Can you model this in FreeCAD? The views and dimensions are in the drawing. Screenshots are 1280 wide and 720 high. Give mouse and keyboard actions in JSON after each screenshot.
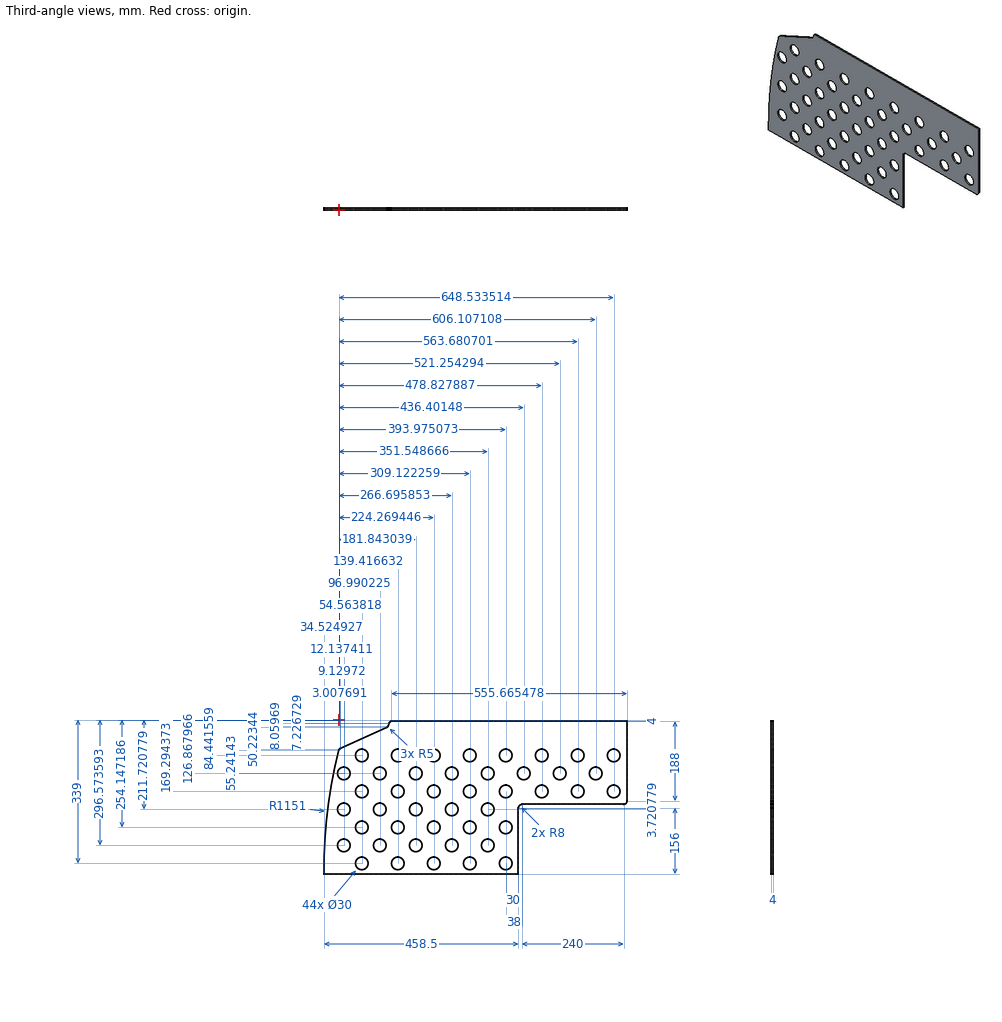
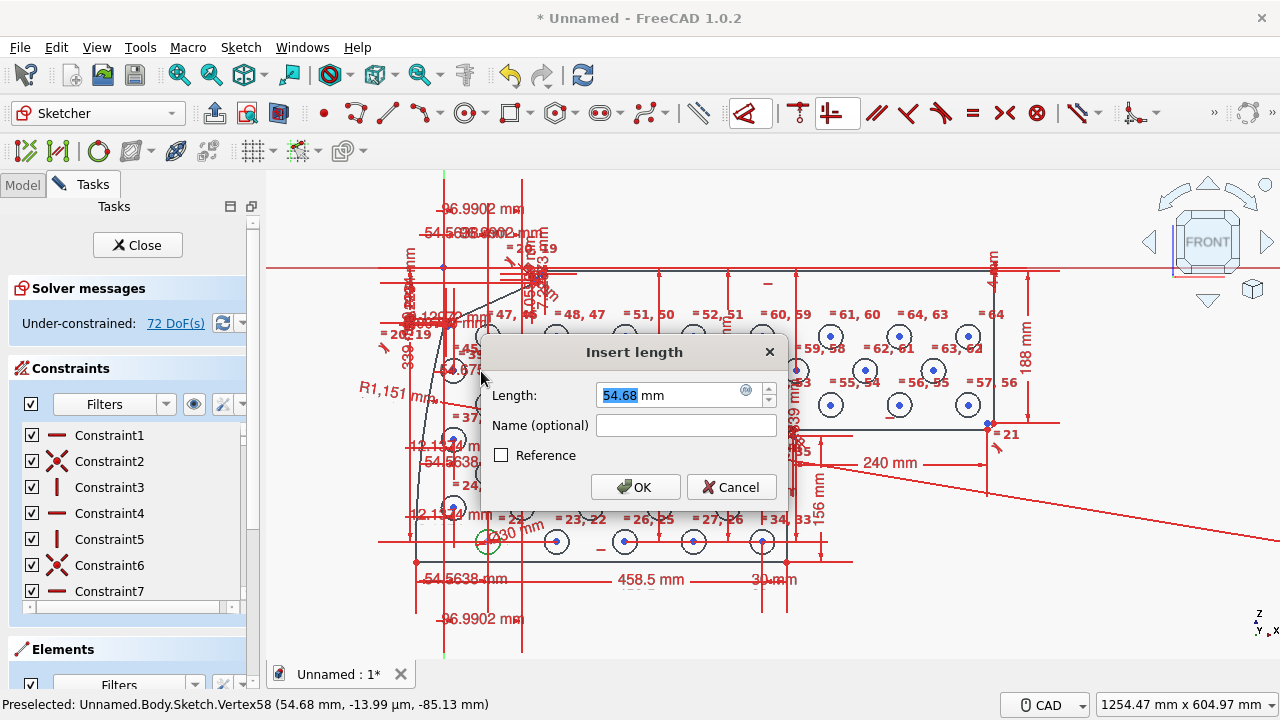
{"action": "type", "text": "54.563818"}
{"action": "key", "text": "Return"}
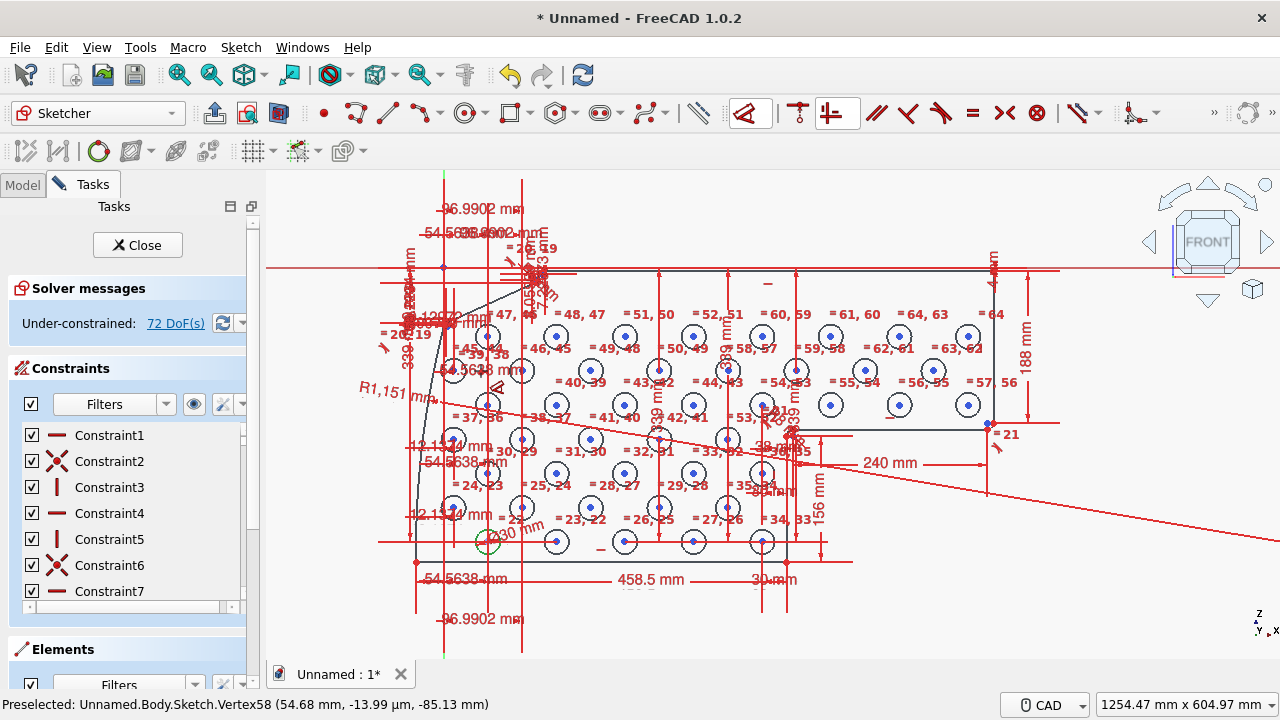
{"action": "left_click", "coordinate": [488, 337]}
{"action": "left_click", "coordinate": [522, 318]}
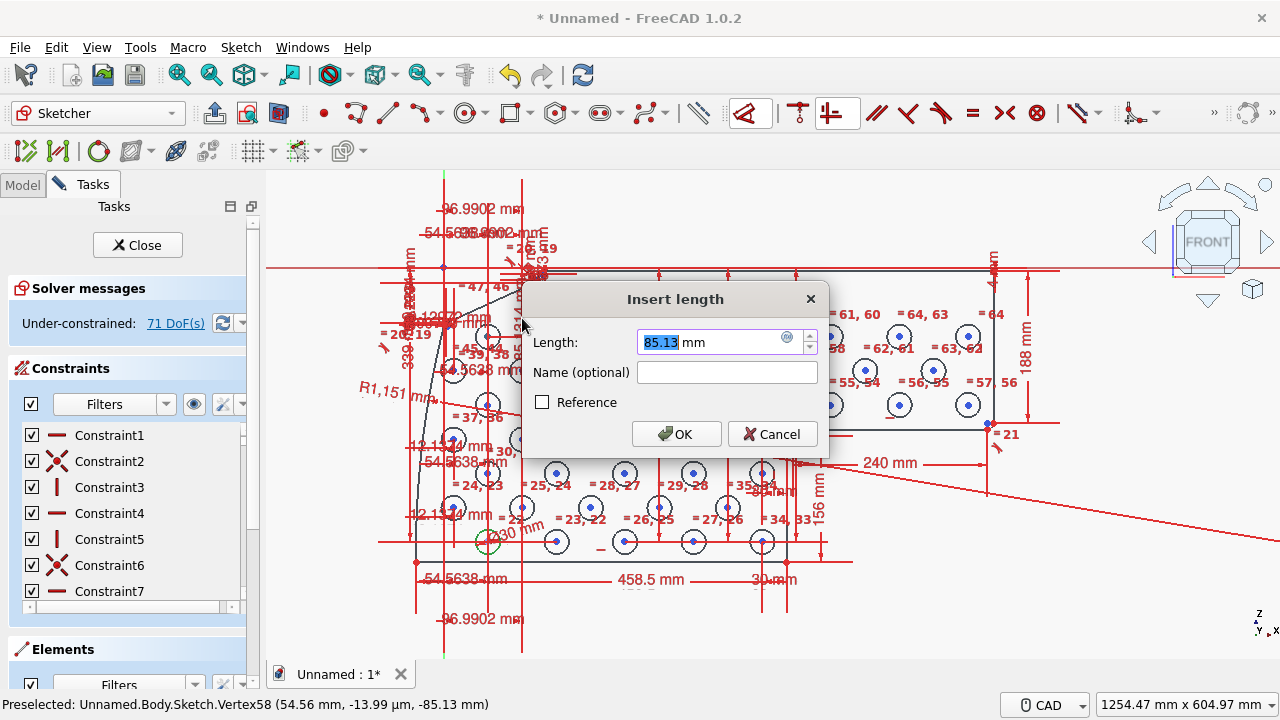
{"action": "type", "text": "84.441559"}
{"action": "key", "text": "Return"}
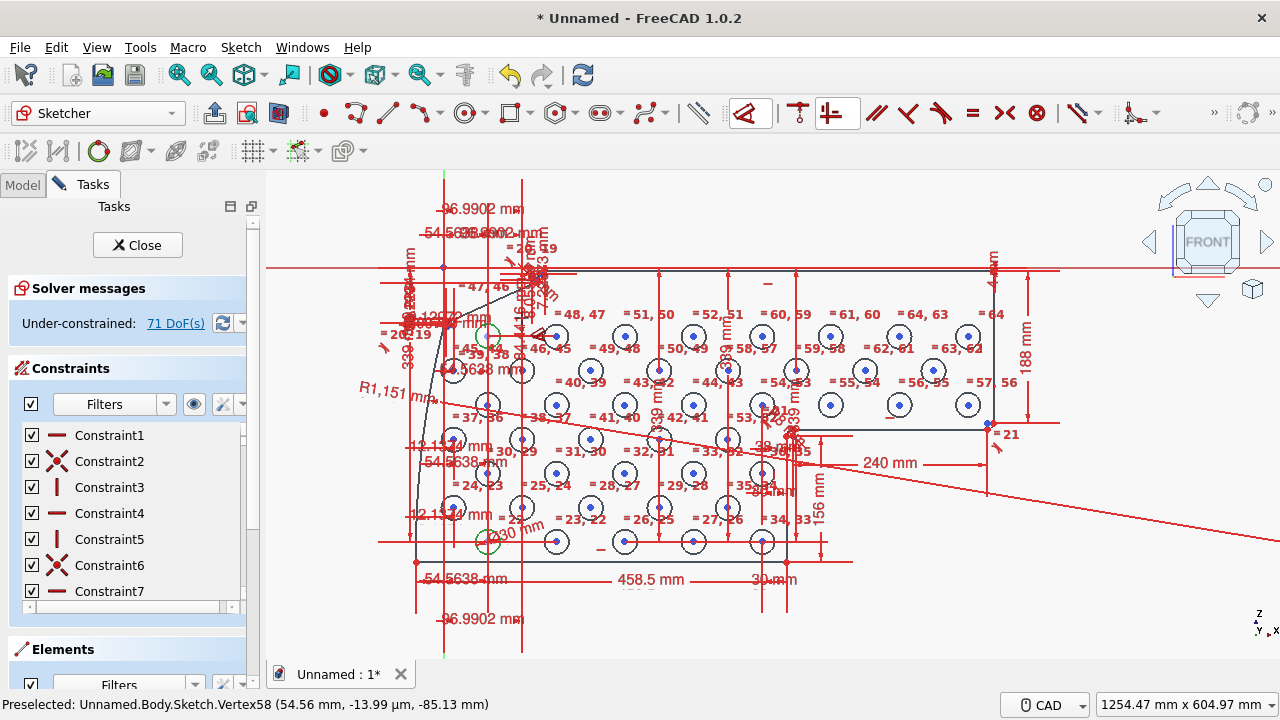
{"action": "left_click", "coordinate": [556, 337]}
{"action": "left_click", "coordinate": [614, 302]}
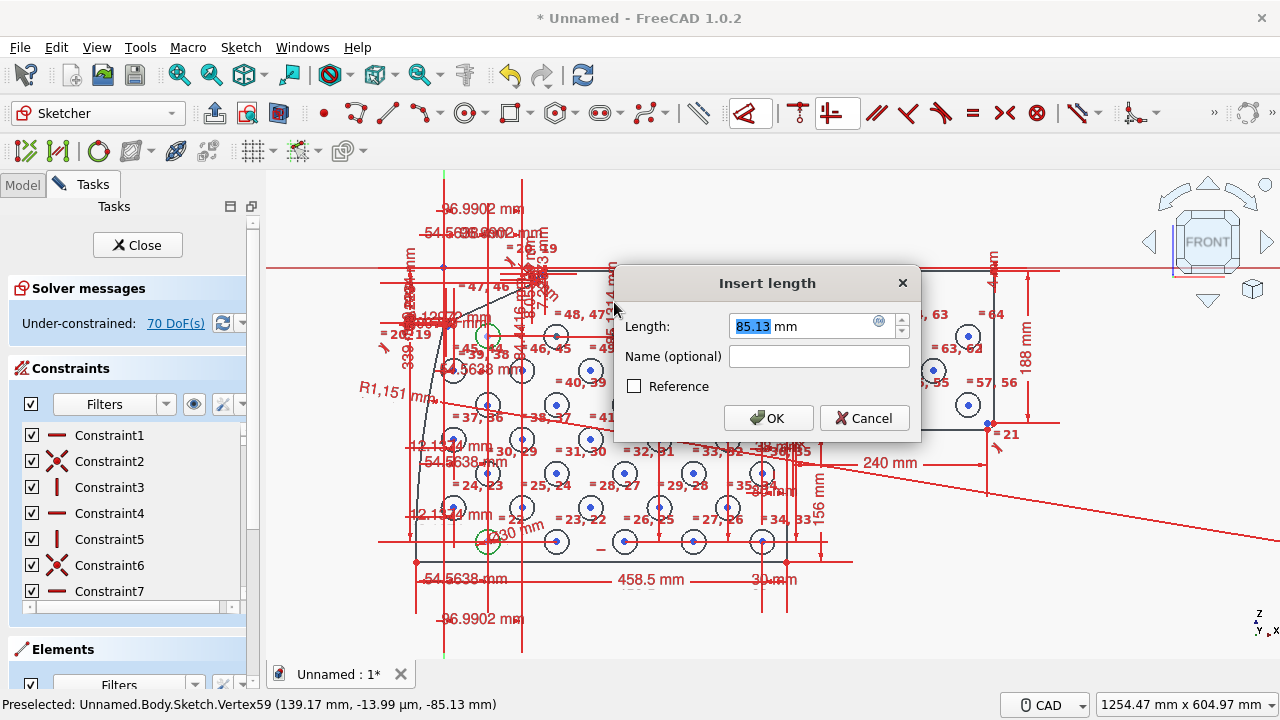
{"action": "type", "text": "84.441559"}
{"action": "key", "text": "Return"}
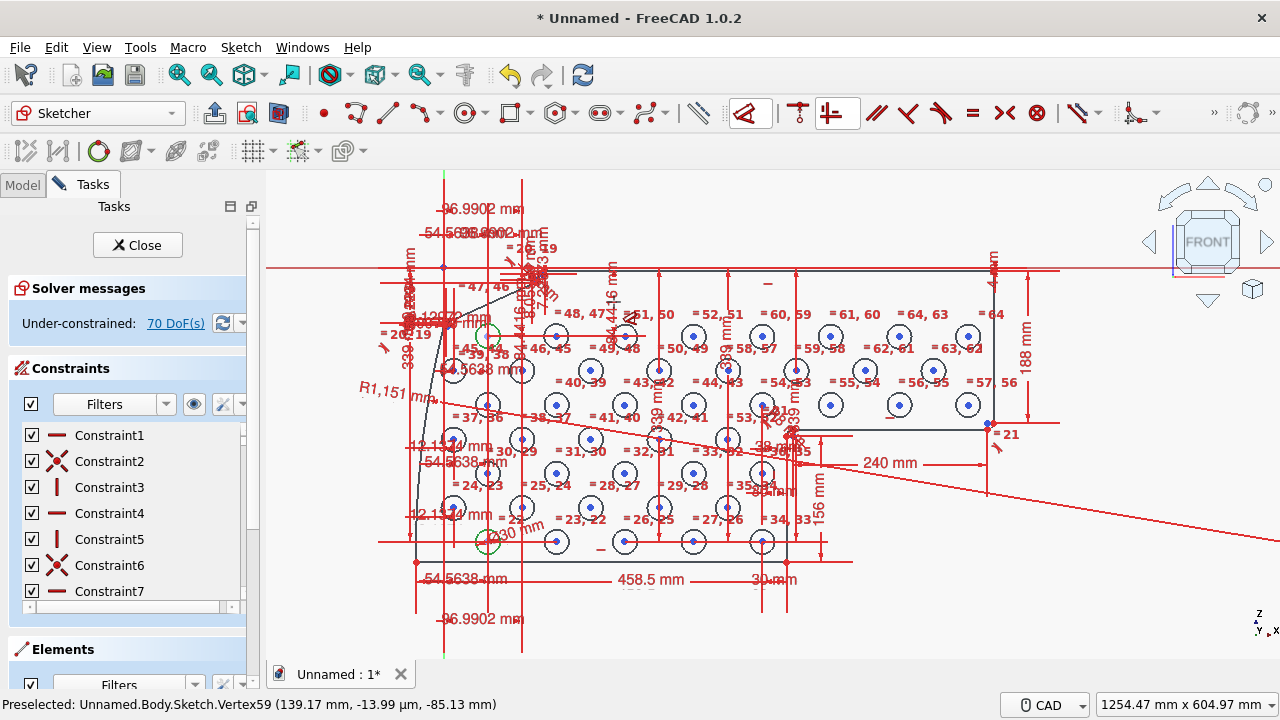
{"action": "left_click", "coordinate": [625, 337]}
{"action": "left_click", "coordinate": [707, 302]}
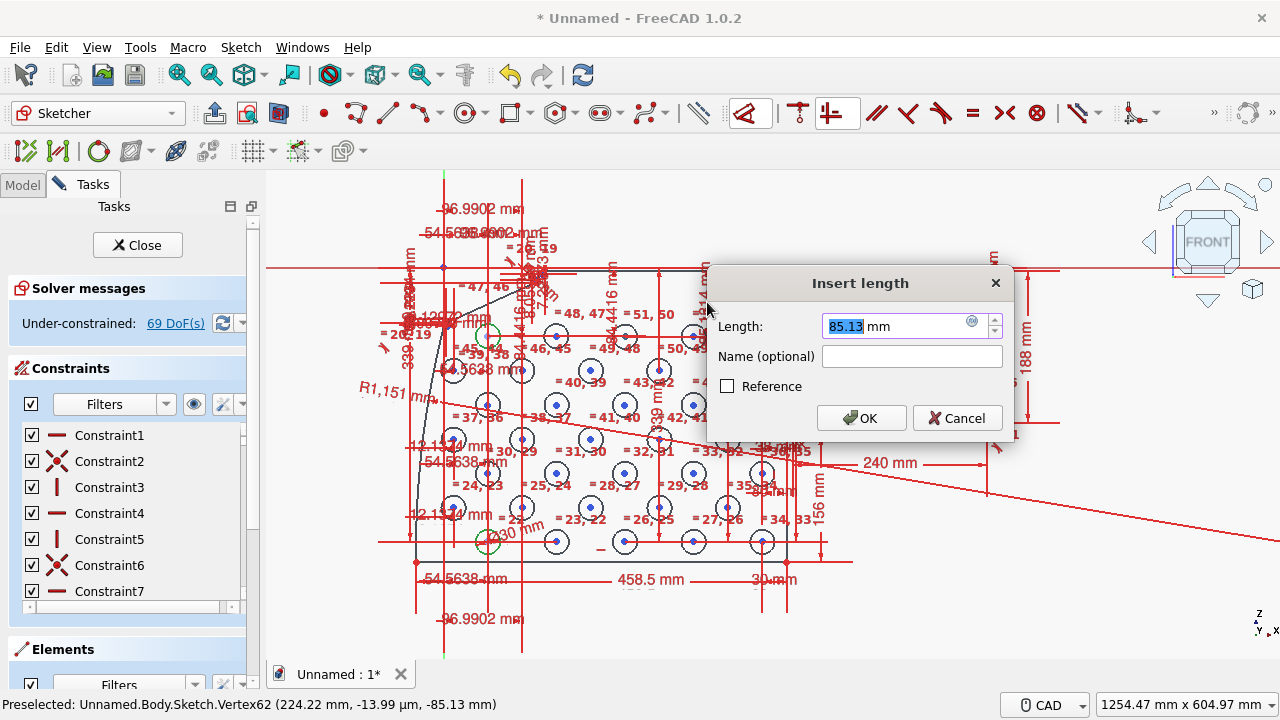
{"action": "type", "text": "84.441559"}
{"action": "key", "text": "Return"}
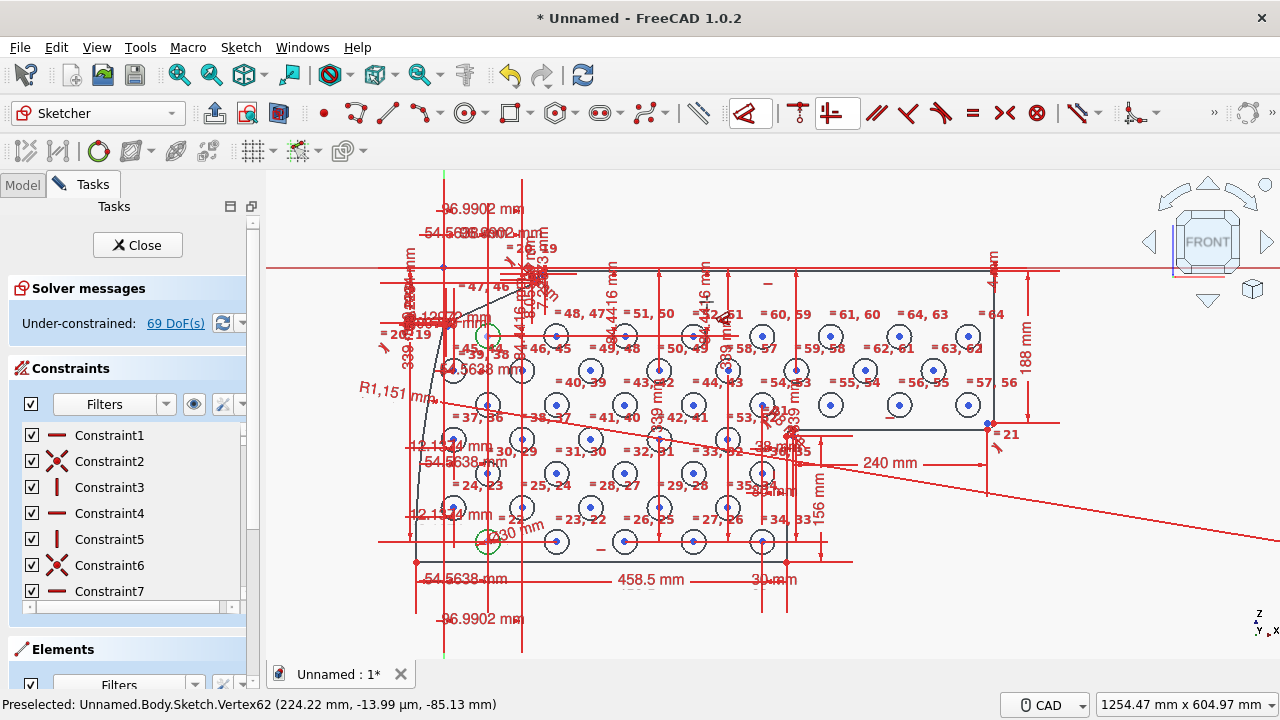
{"action": "left_click", "coordinate": [694, 337]}
{"action": "left_click", "coordinate": [338, 302]}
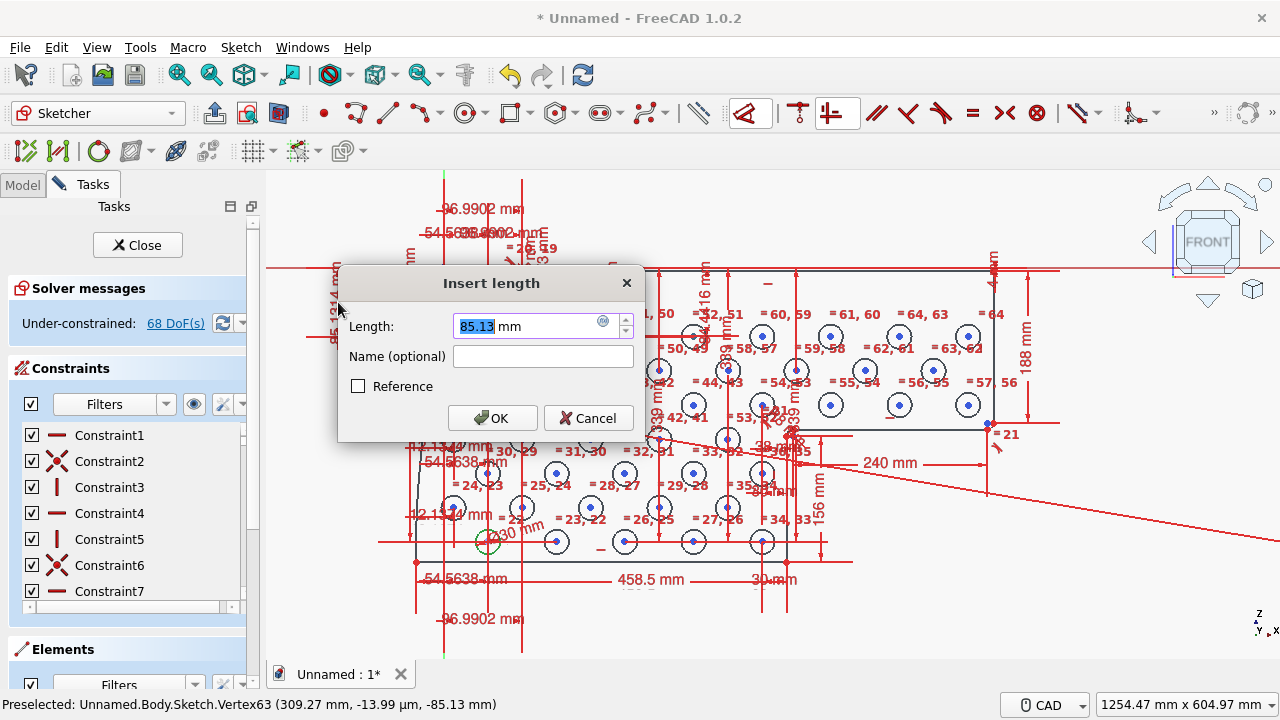
{"action": "type", "text": "84.441559"}
{"action": "key", "text": "Return"}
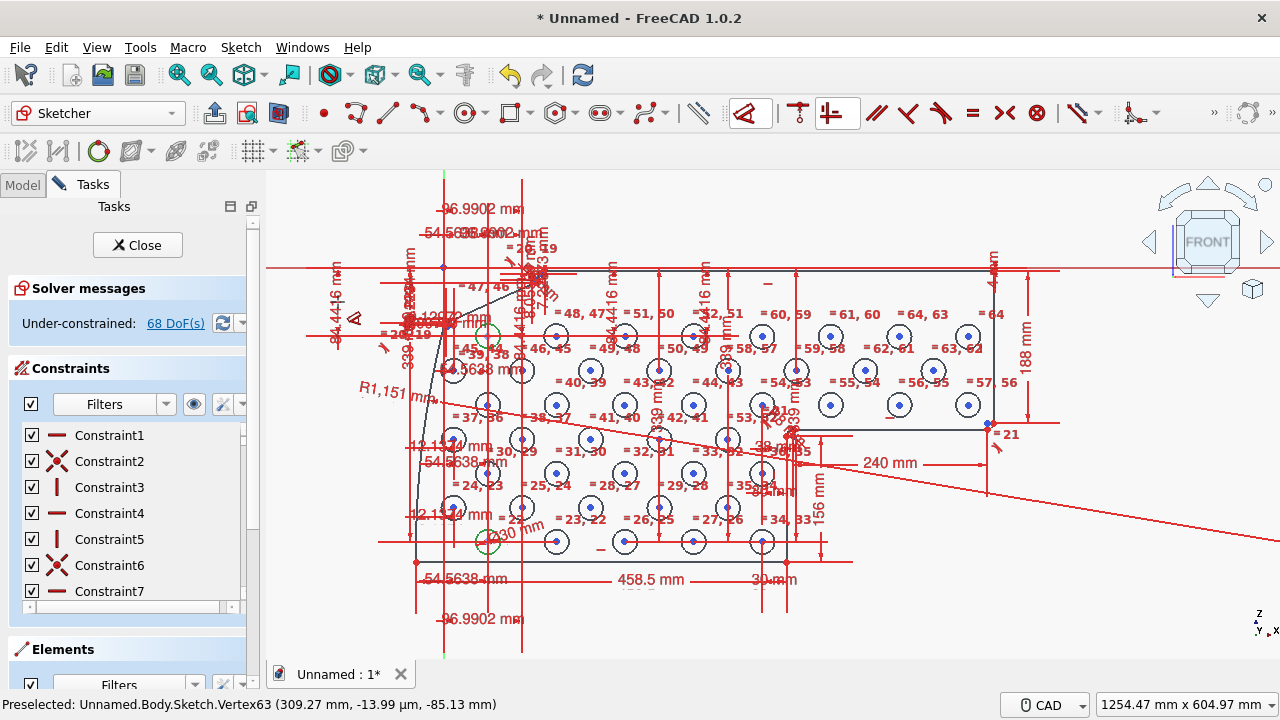
{"action": "left_click", "coordinate": [797, 371]}
{"action": "left_click", "coordinate": [620, 234]}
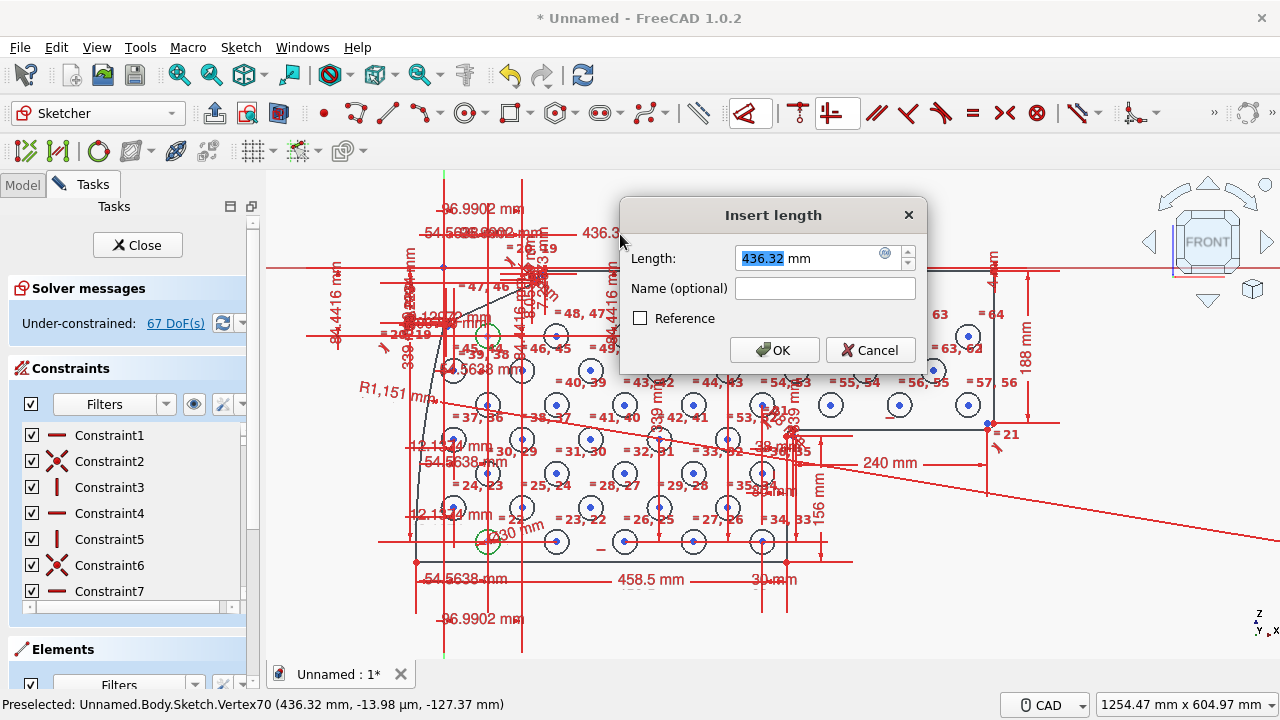
{"action": "type", "text": "436.40148"}
{"action": "key", "text": "Return"}